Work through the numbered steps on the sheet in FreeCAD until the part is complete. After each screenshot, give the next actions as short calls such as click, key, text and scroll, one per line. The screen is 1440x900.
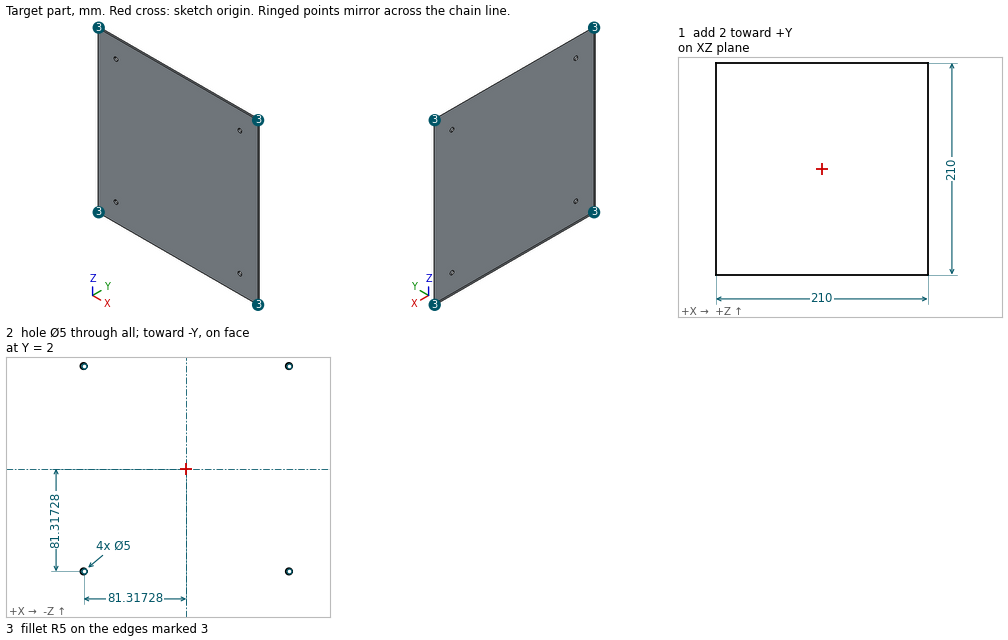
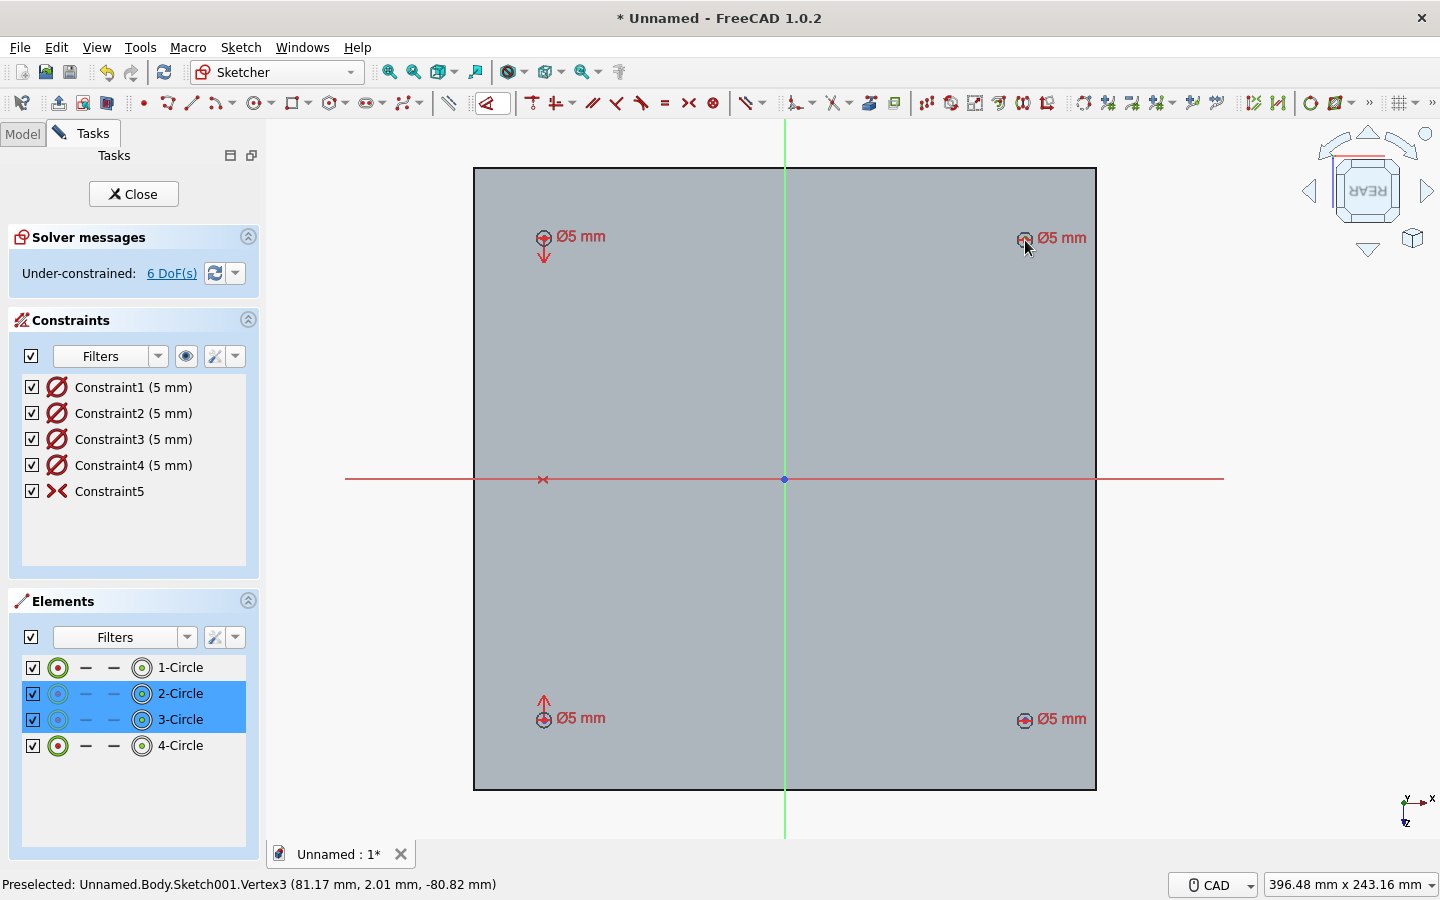
click(785, 764)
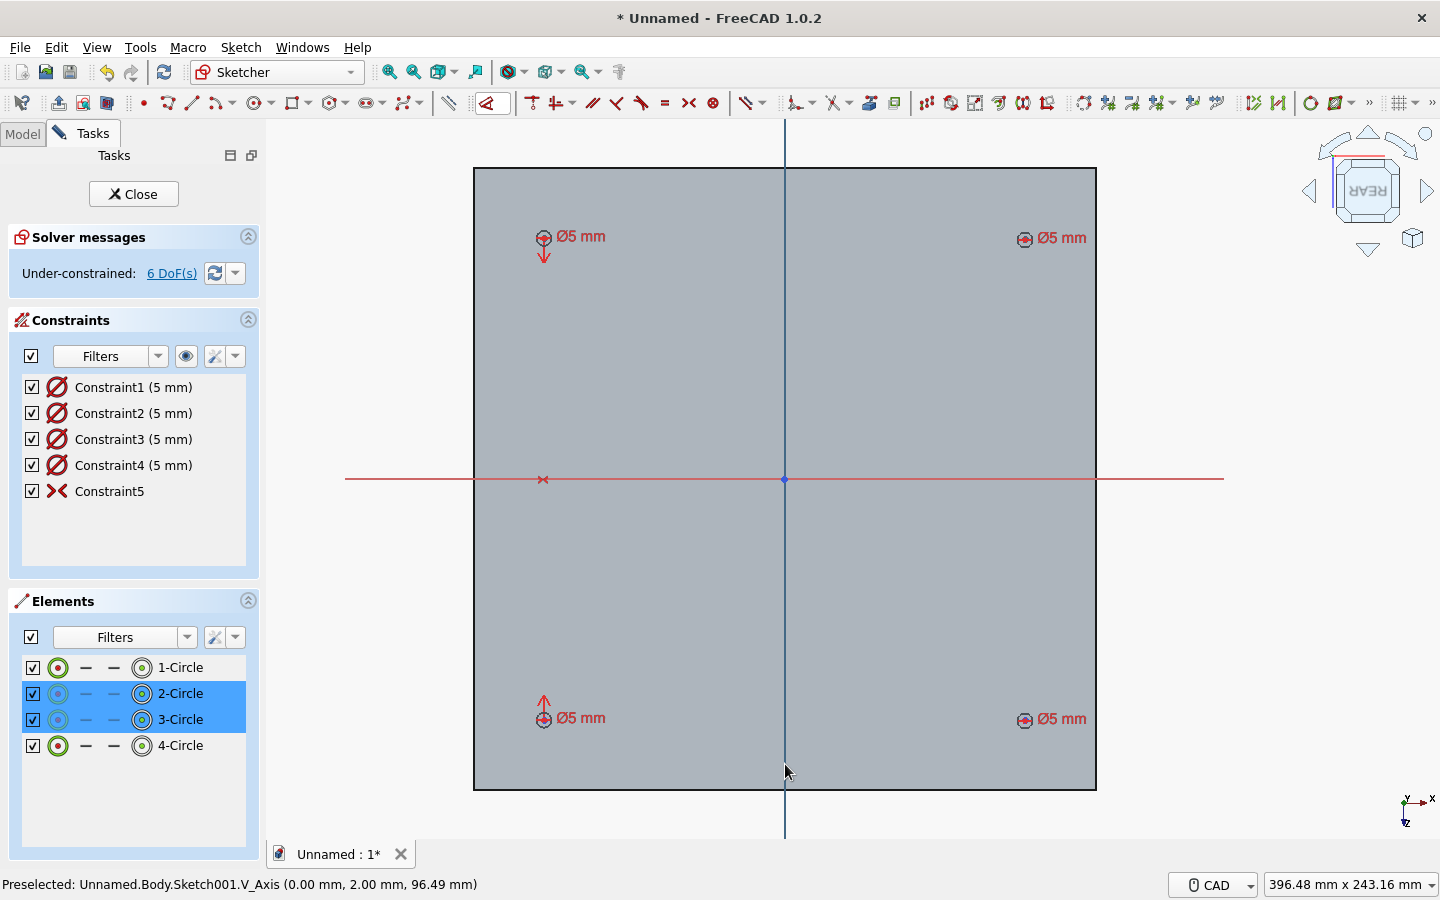
click(690, 104)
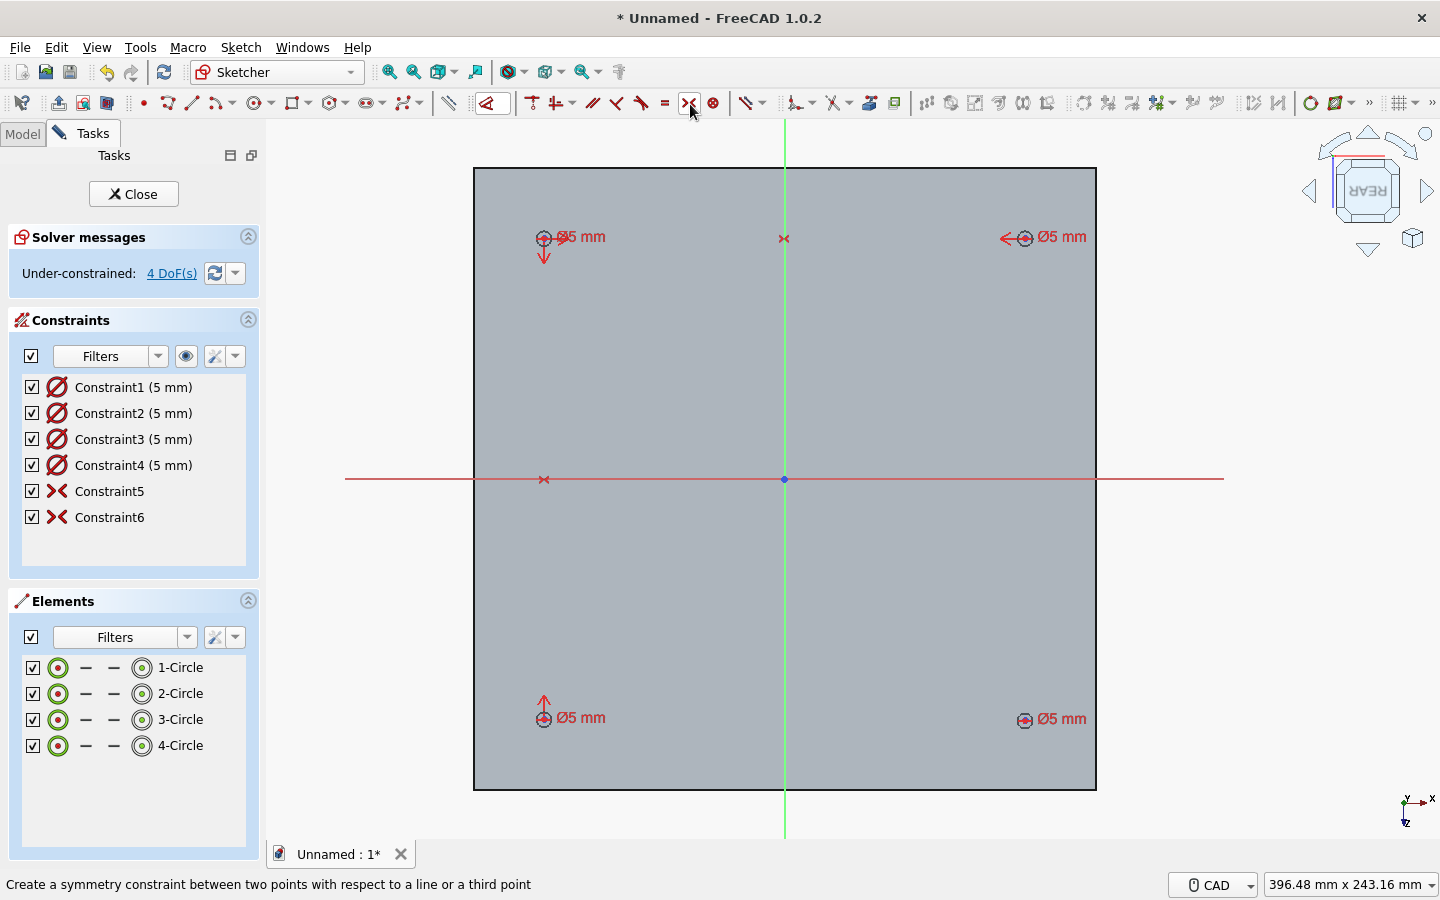
click(544, 720)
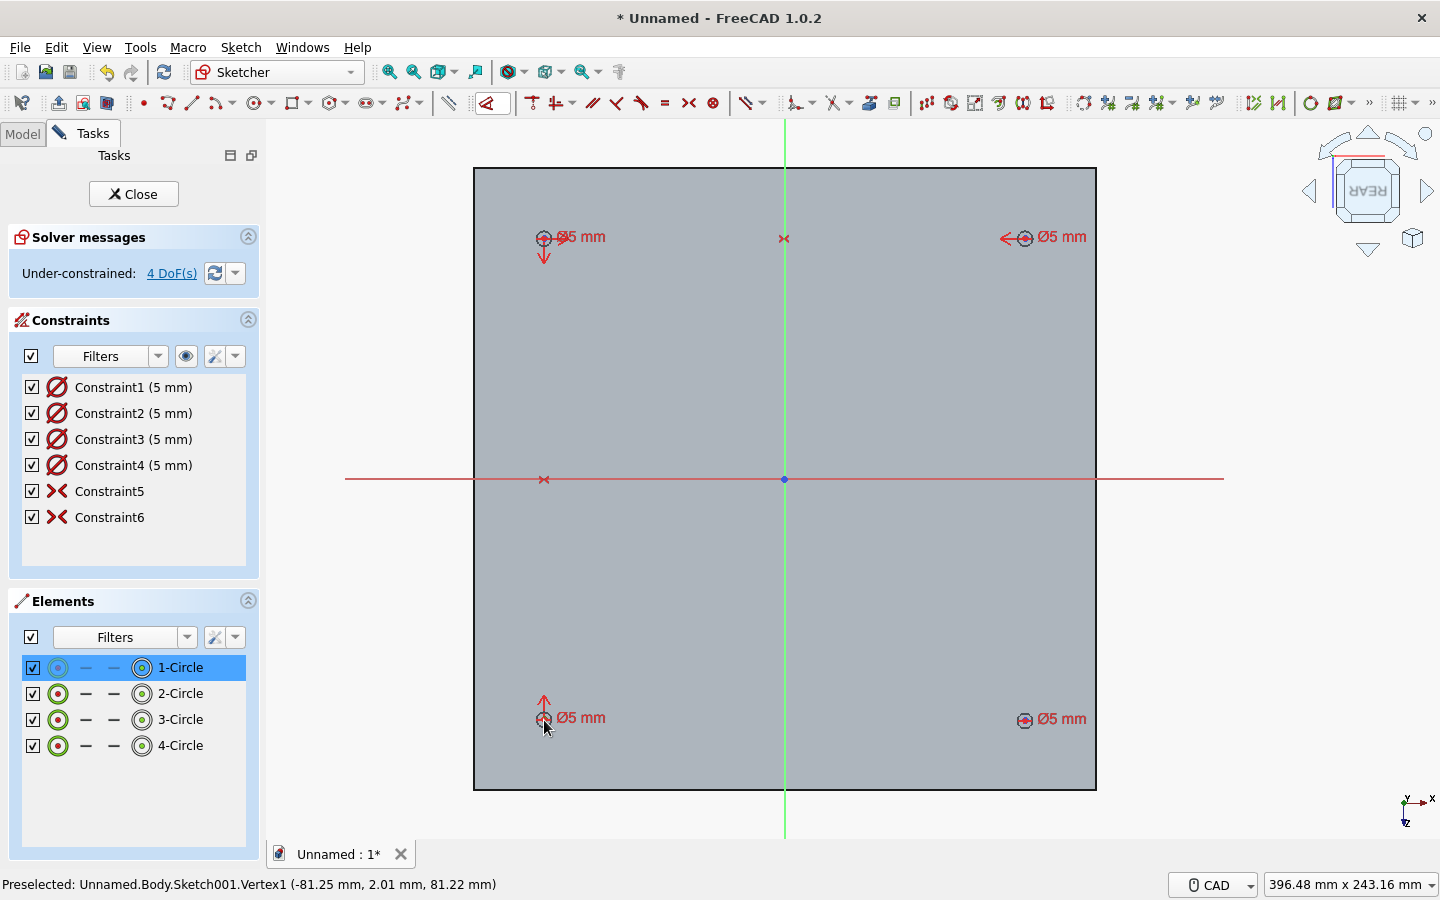
click(1025, 721)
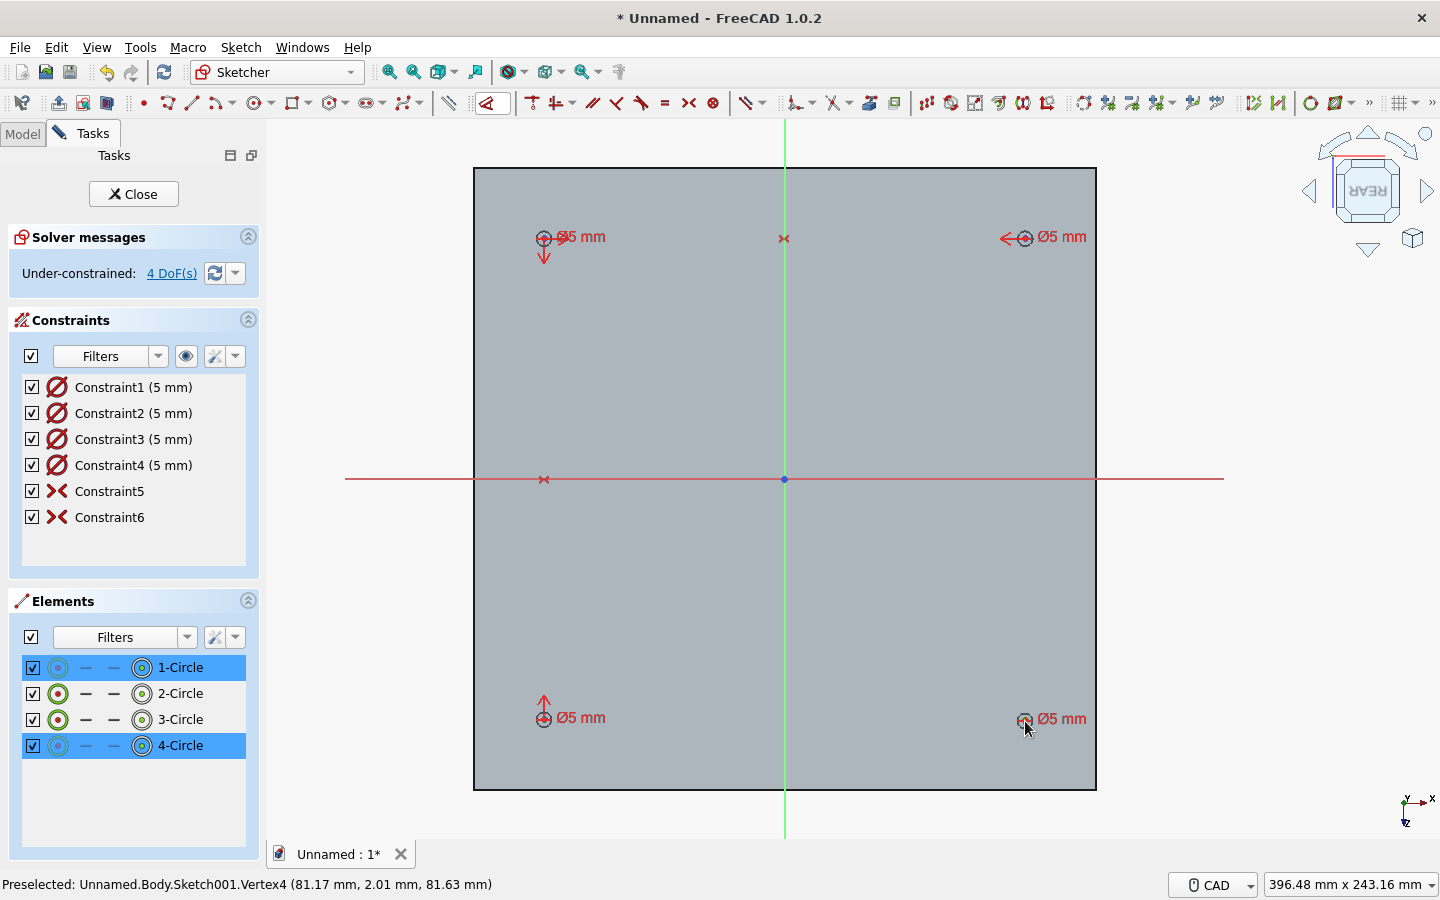
click(785, 764)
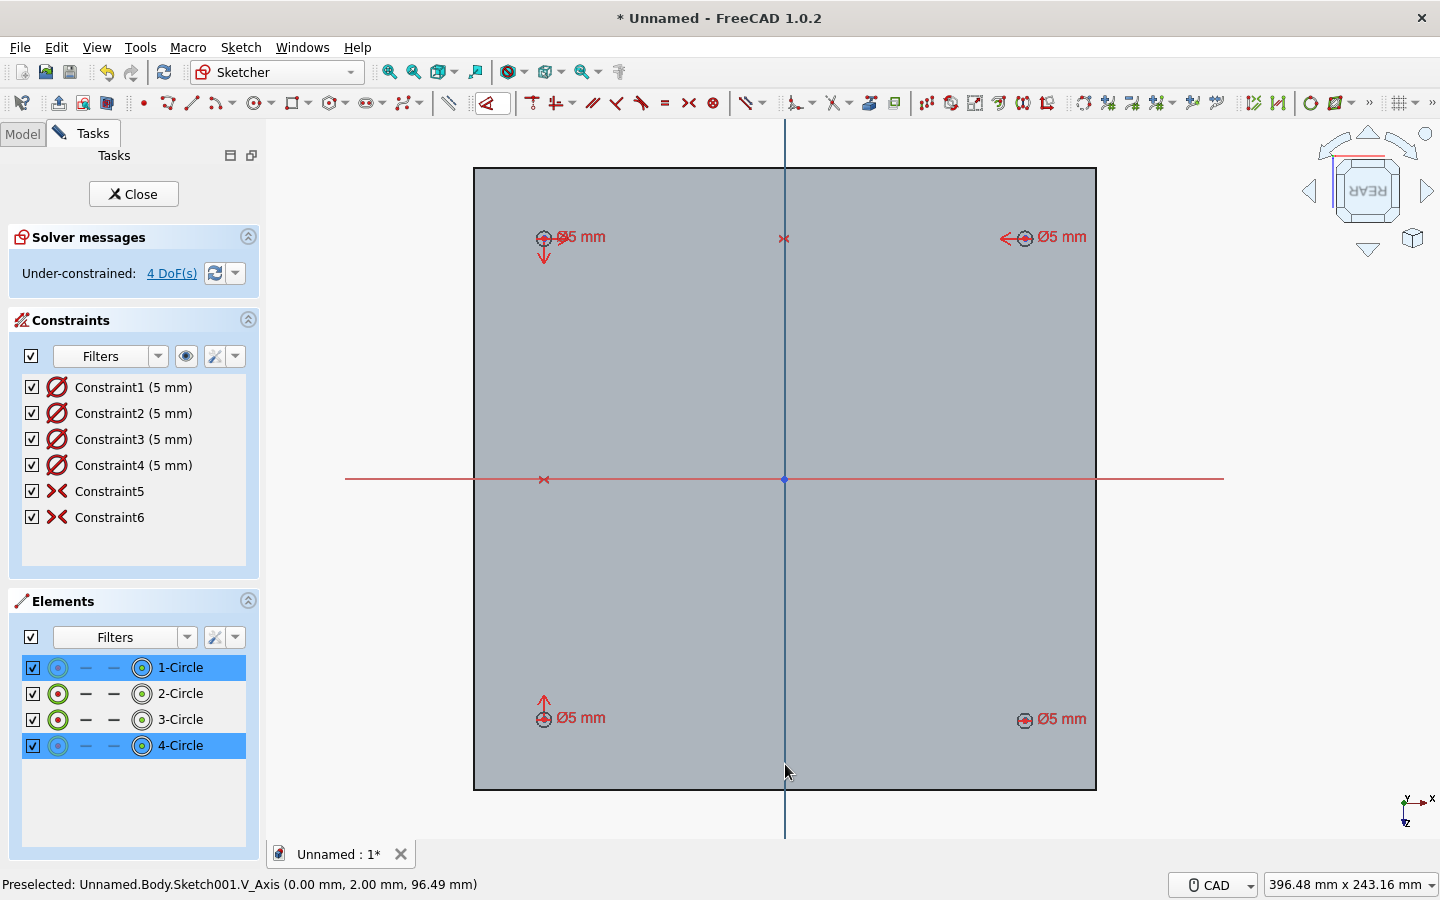
click(690, 104)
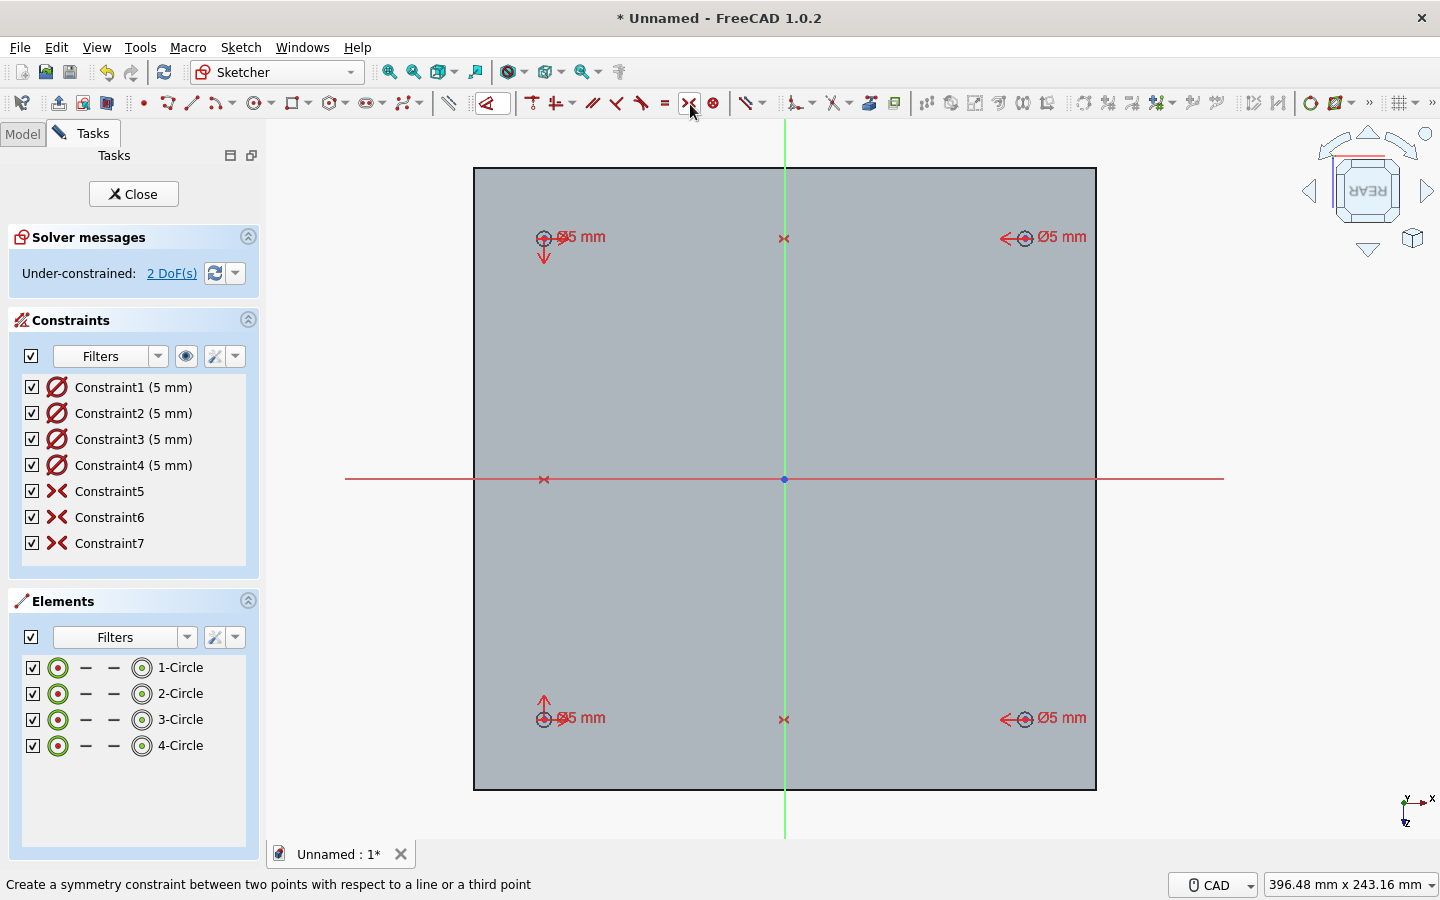
click(486, 104)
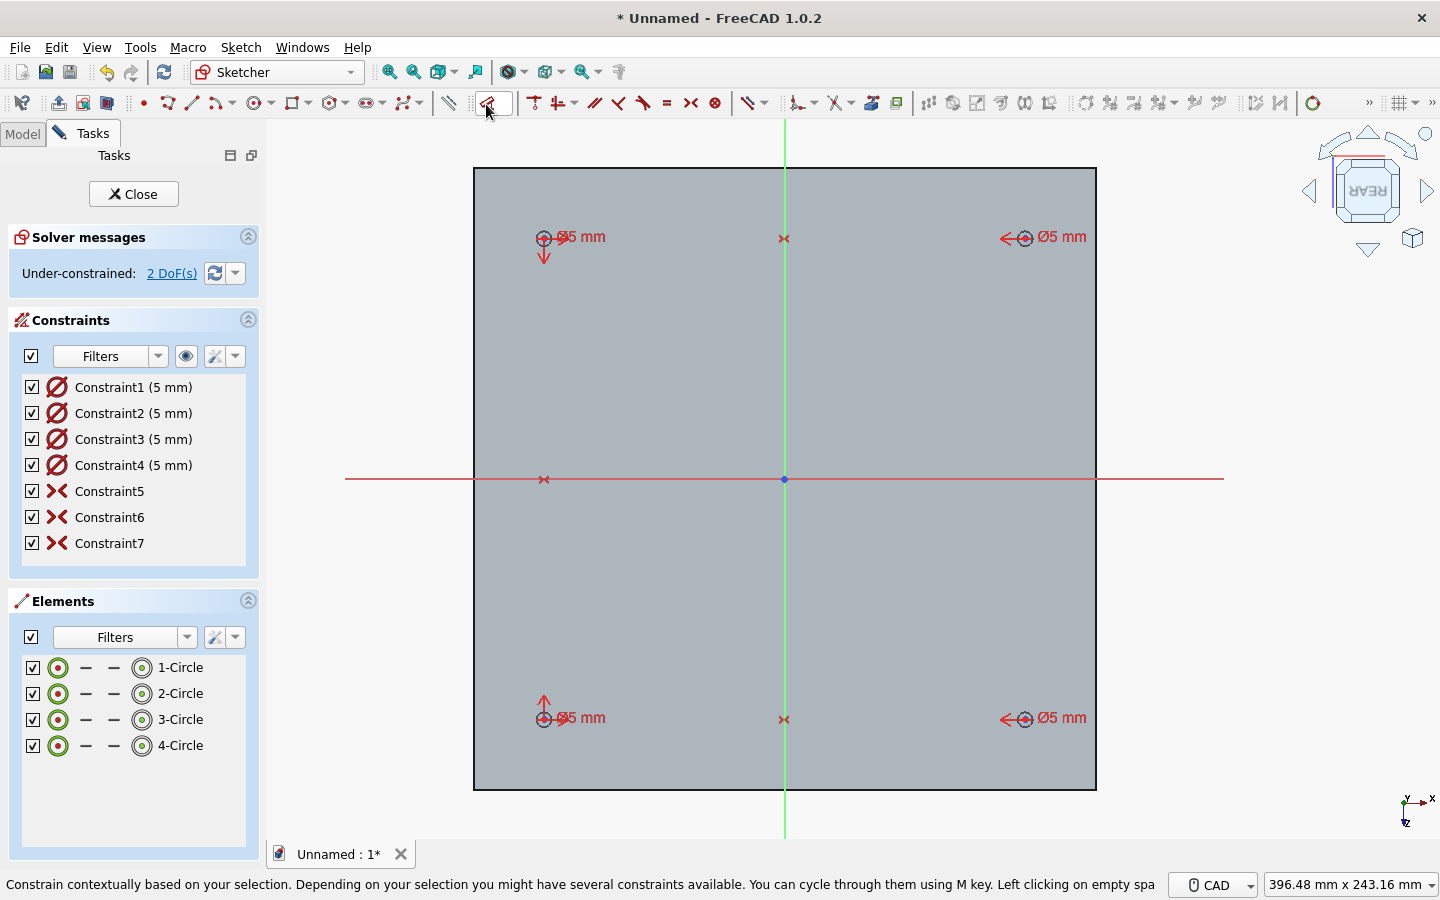
click(544, 720)
click(664, 754)